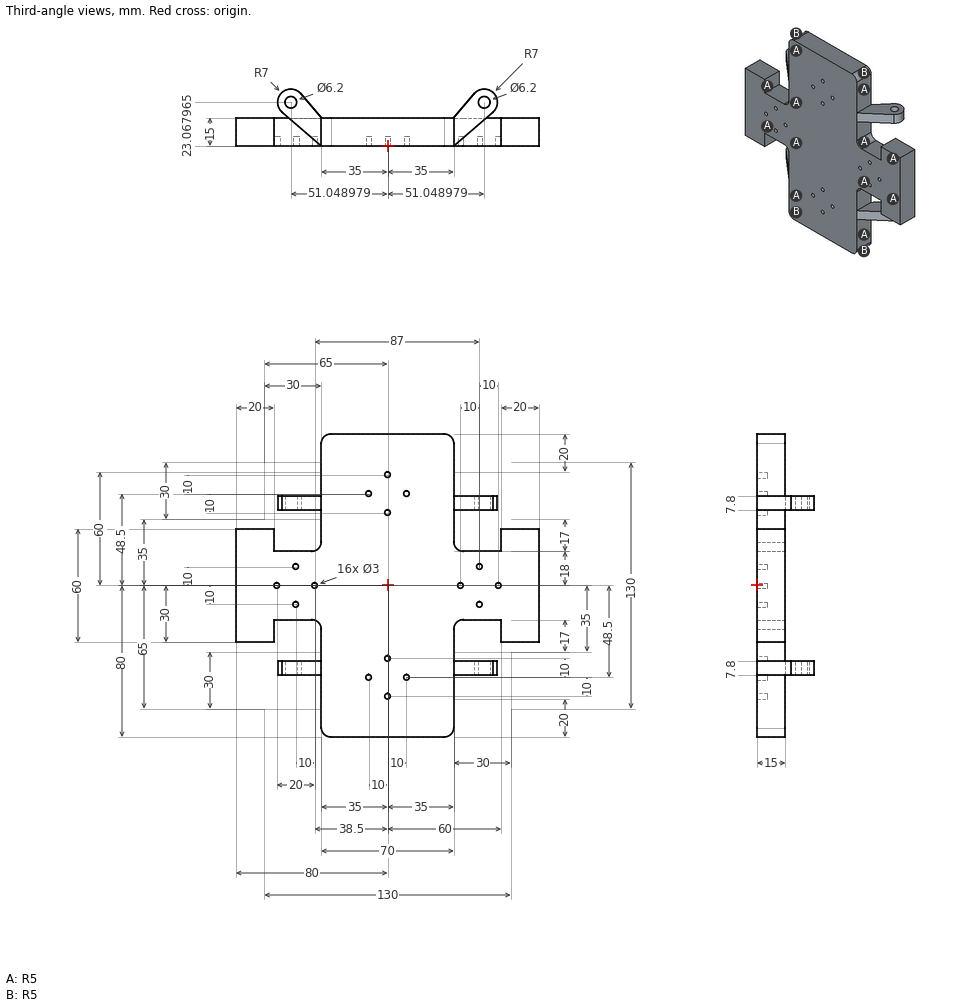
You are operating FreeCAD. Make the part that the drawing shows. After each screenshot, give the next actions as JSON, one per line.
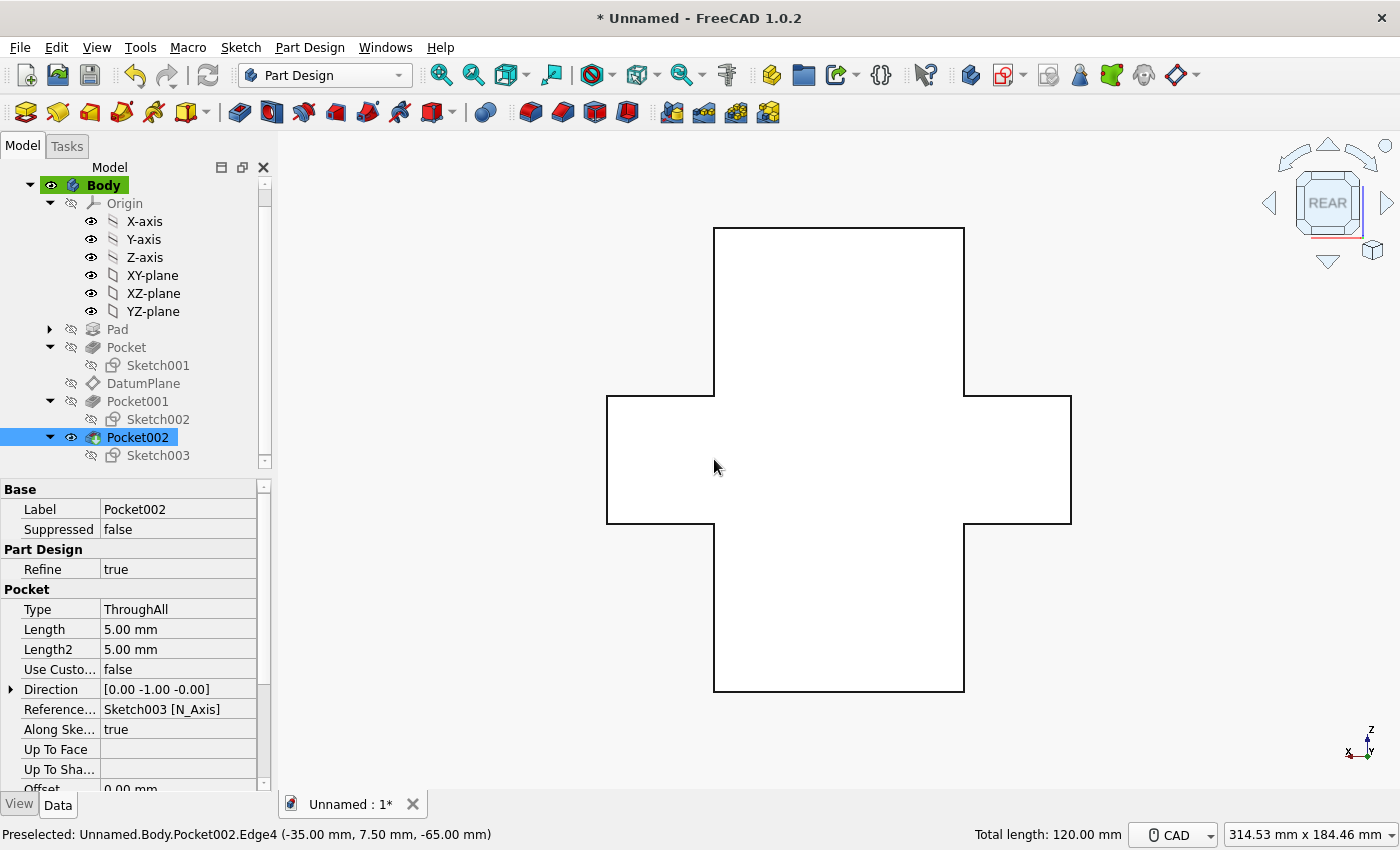
{"action": "key", "text": "6"}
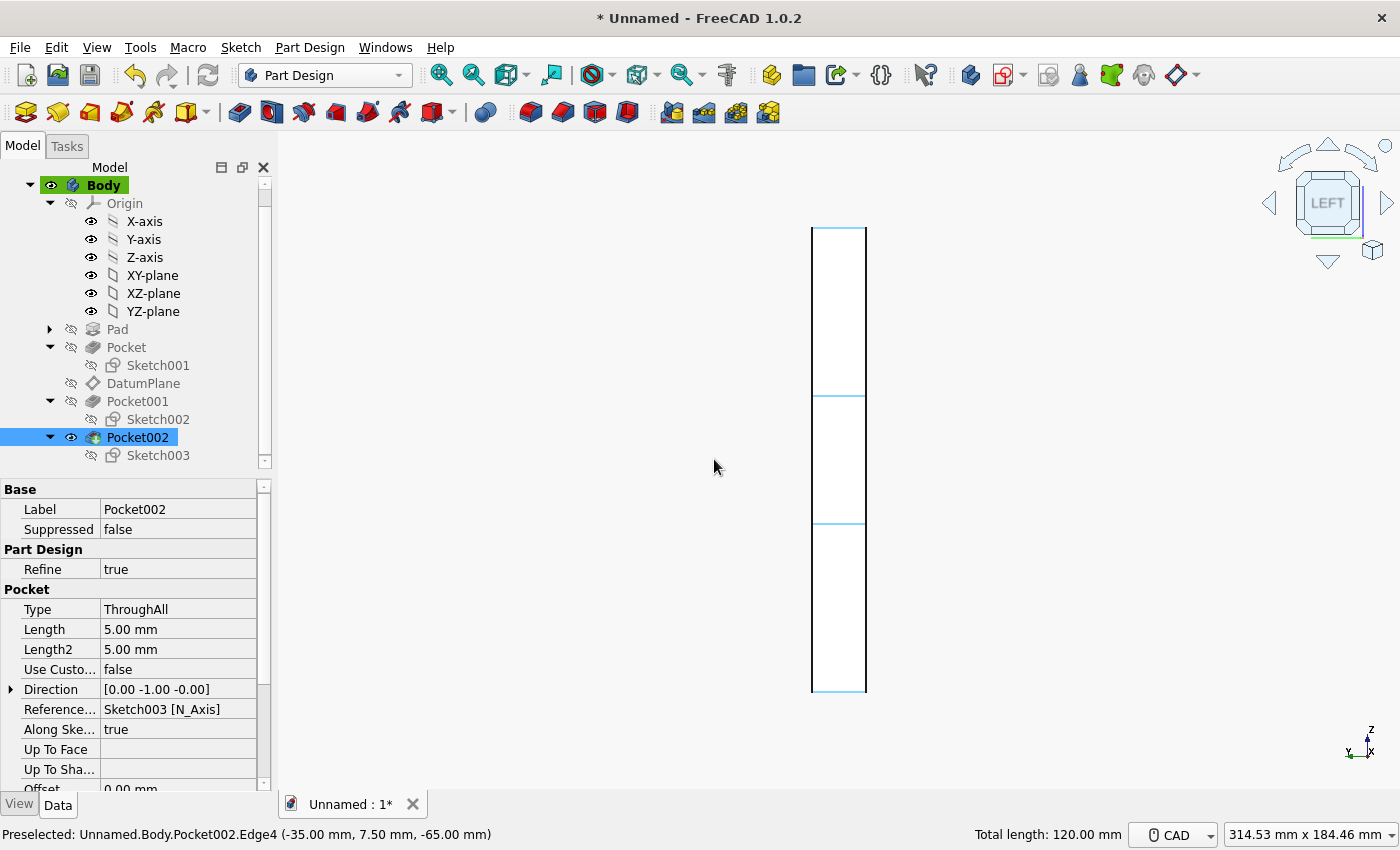
{"action": "key", "text": "v 3"}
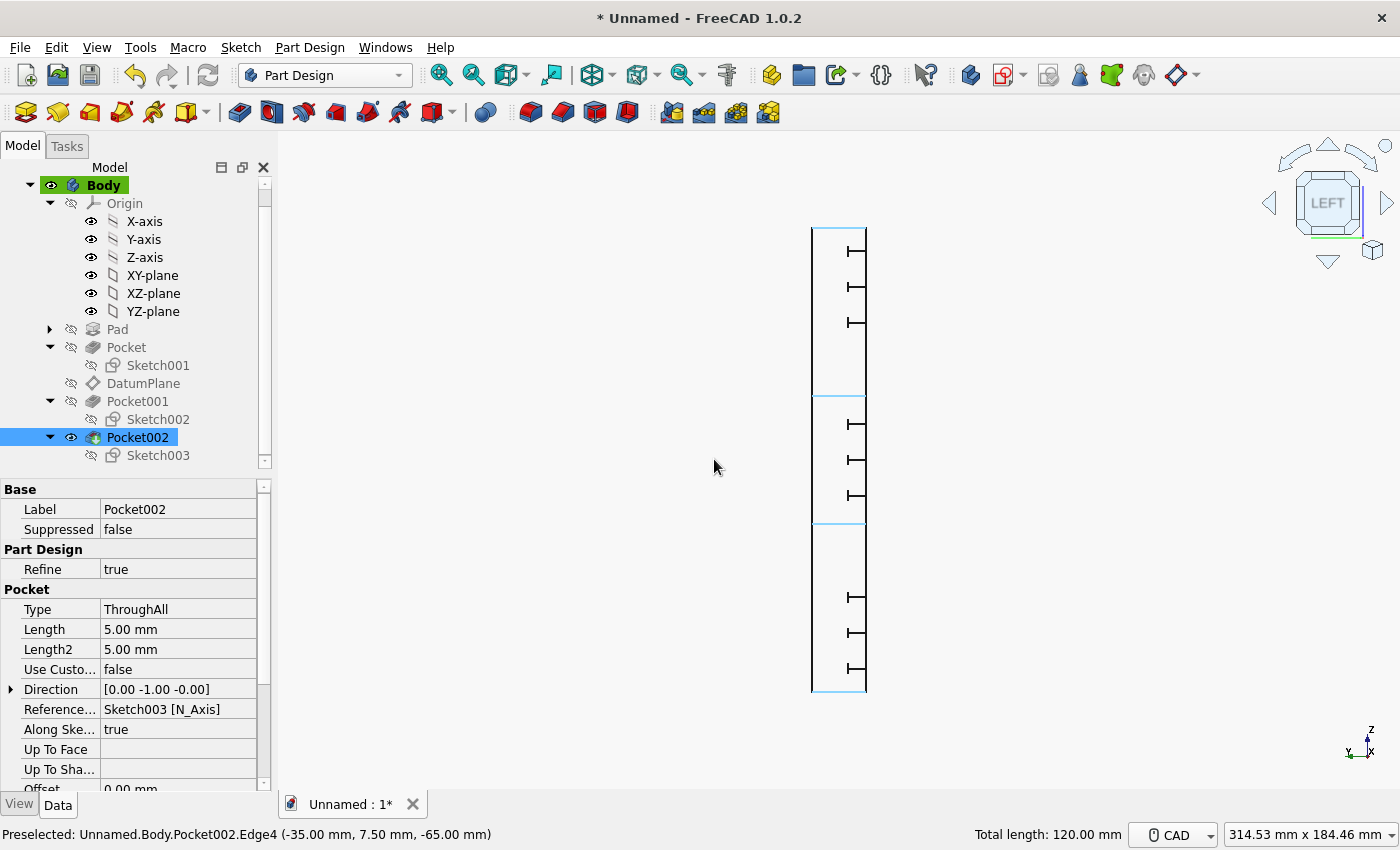
{"action": "key", "text": "0"}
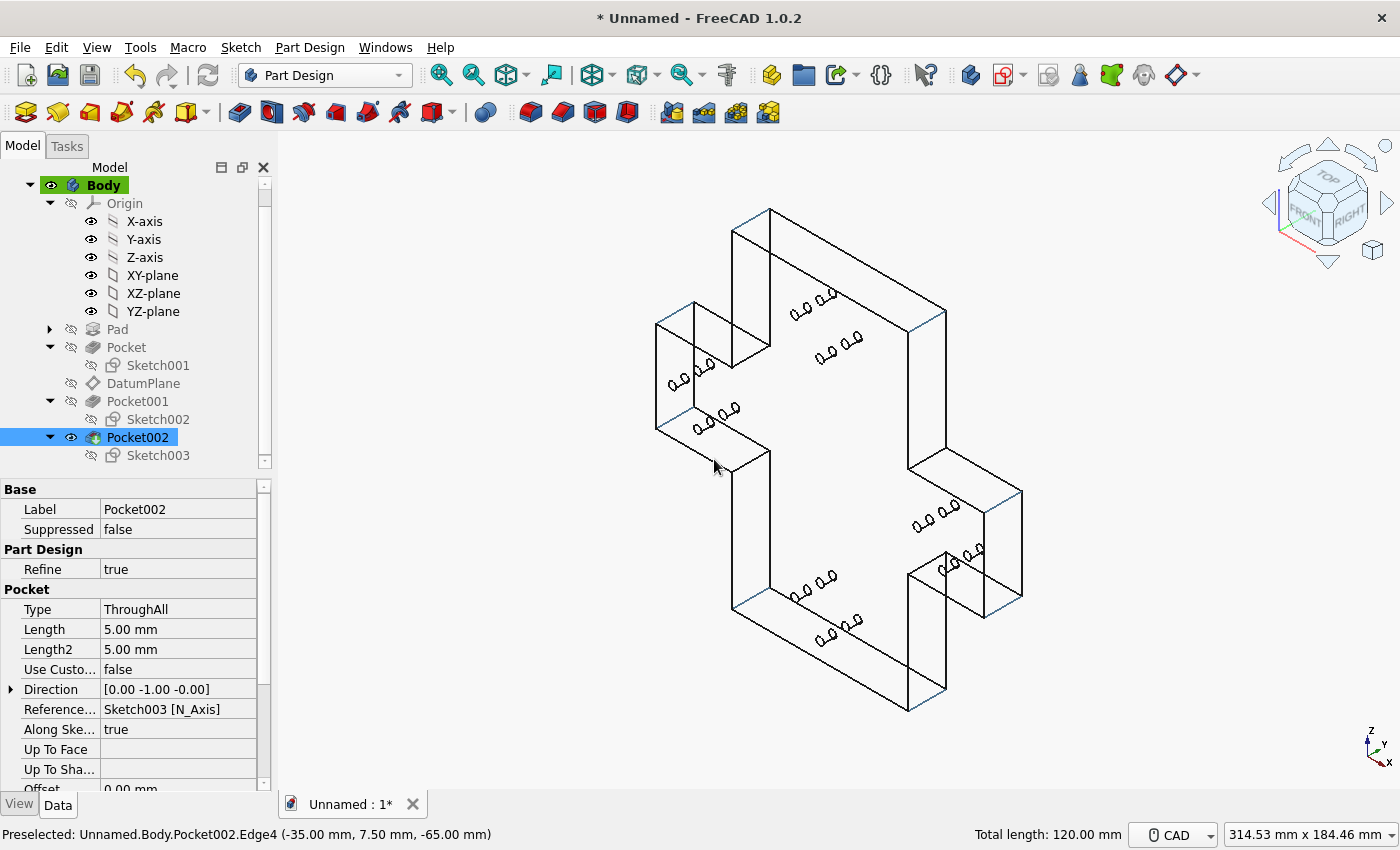
{"action": "left_click", "coordinate": [927, 458], "text": "ctrl"}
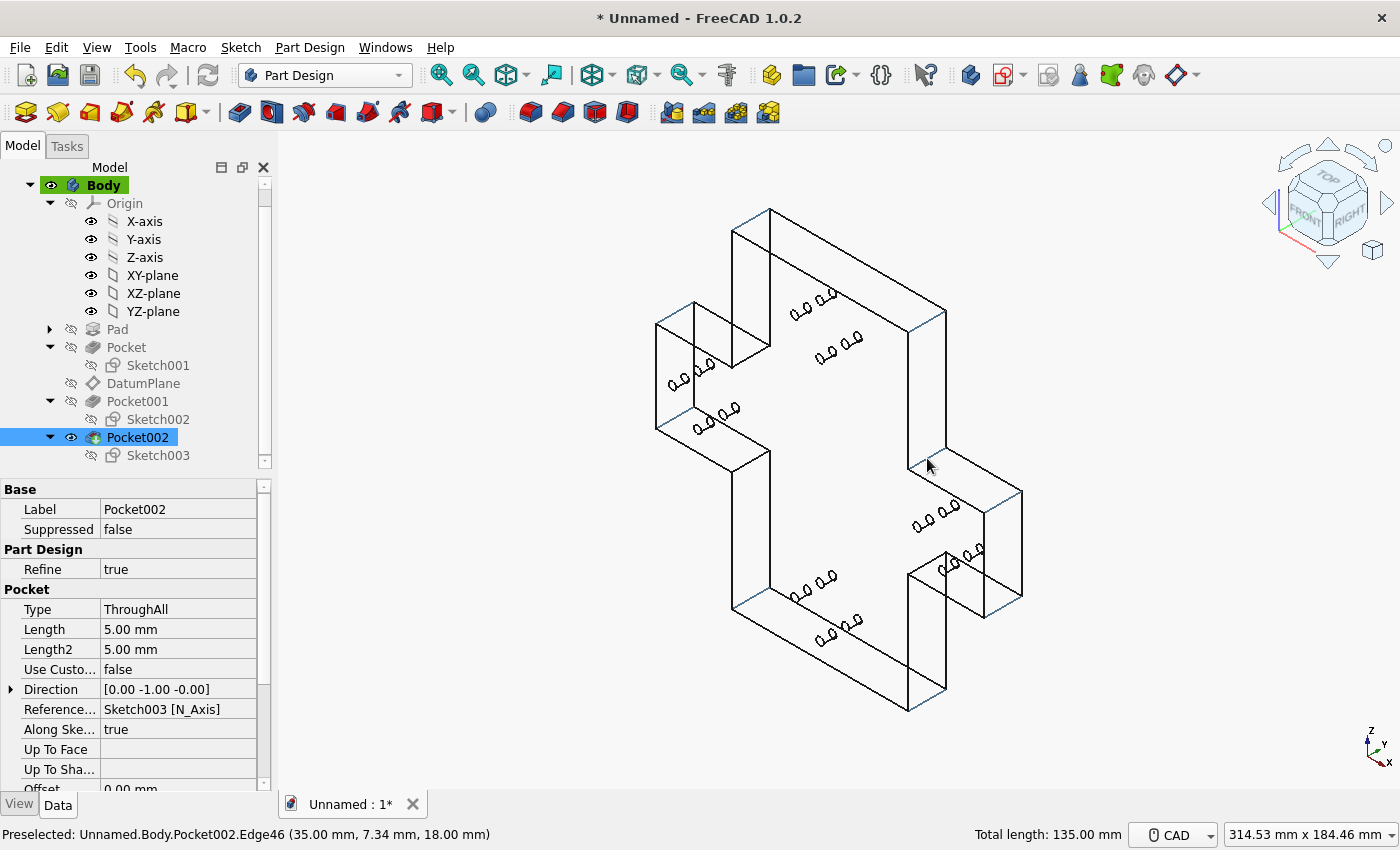
{"action": "left_click", "coordinate": [751, 460], "text": "ctrl"}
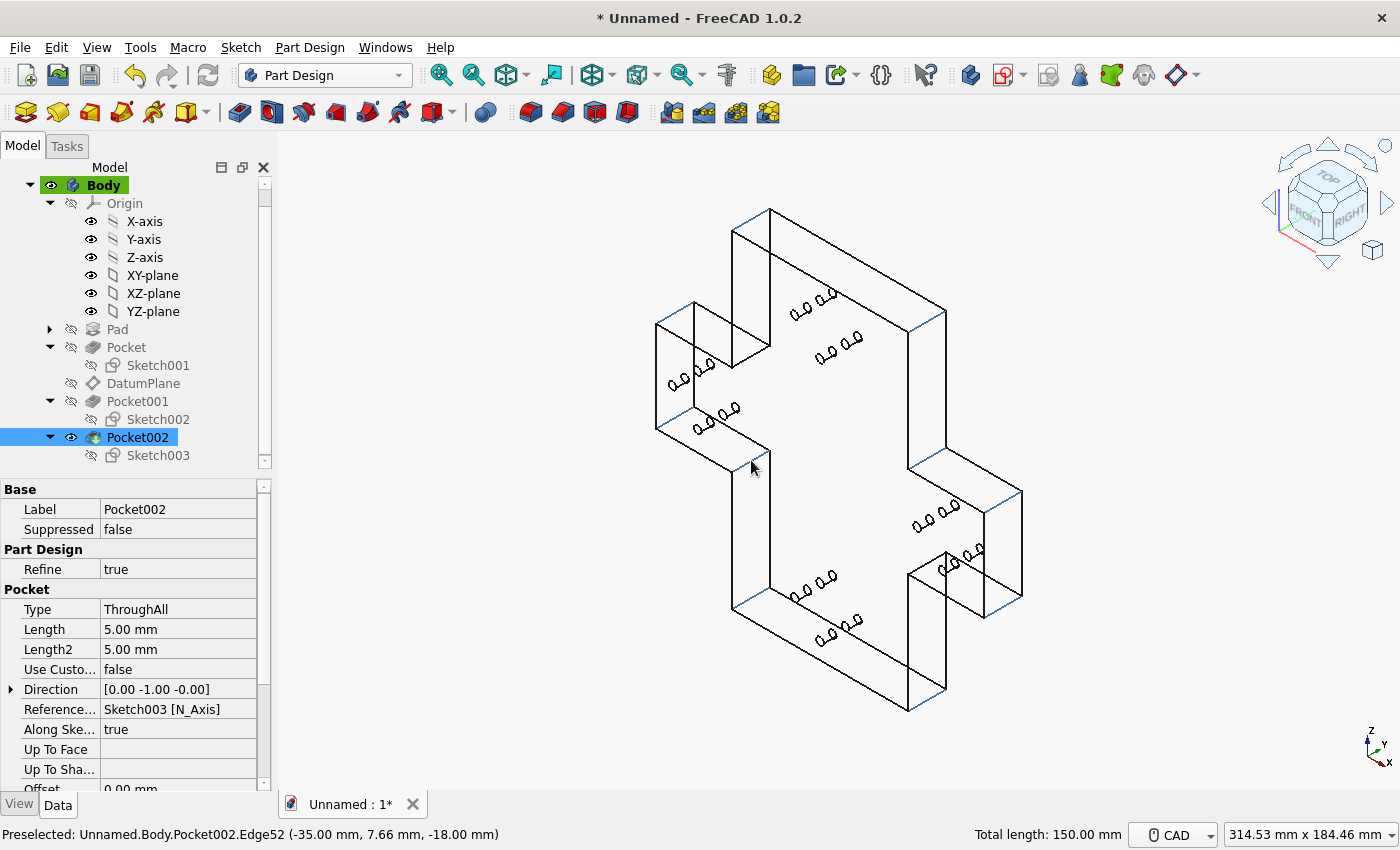
{"action": "left_click", "coordinate": [751, 356], "text": "ctrl"}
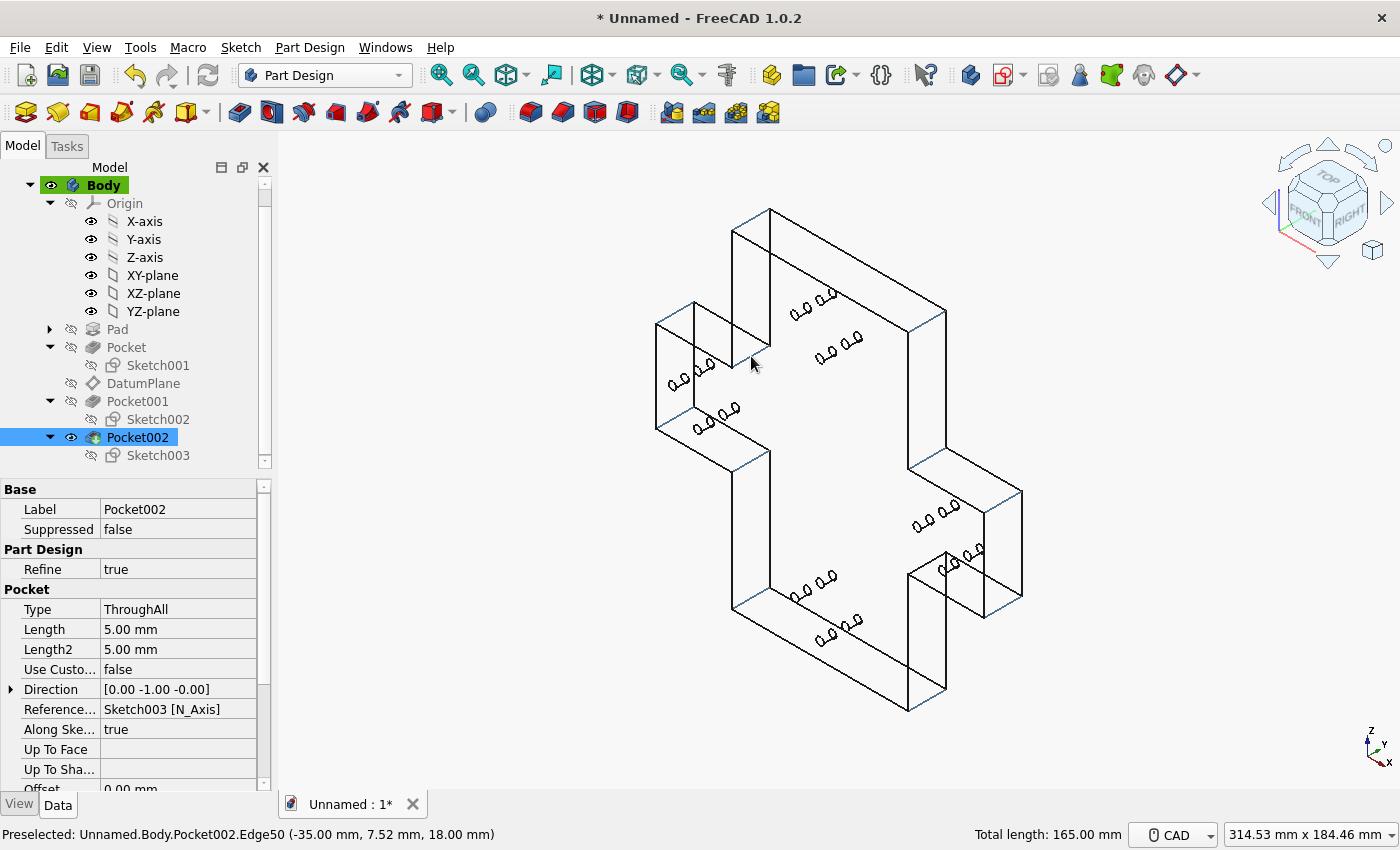
{"action": "left_click", "coordinate": [927, 562], "text": "ctrl"}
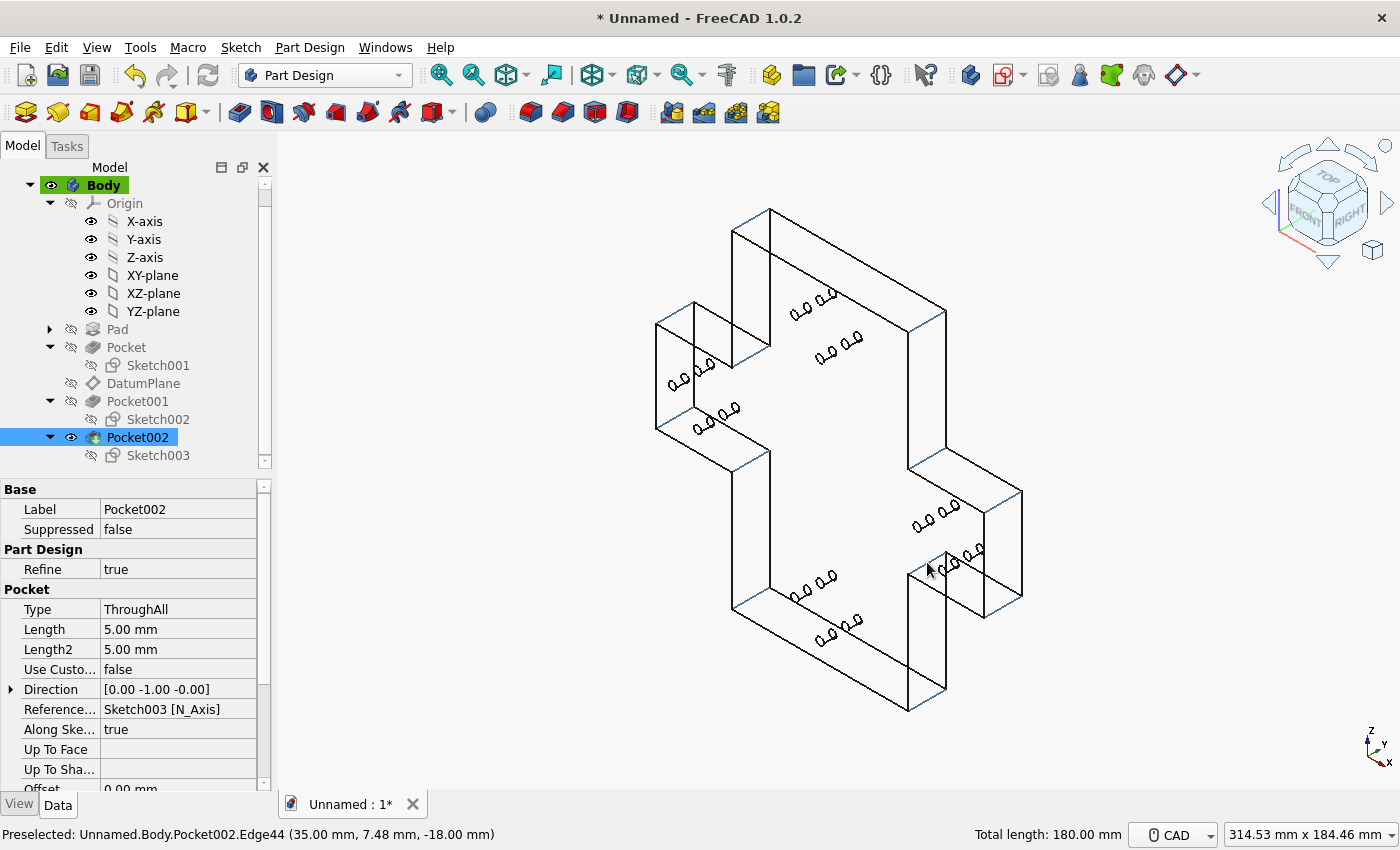
{"action": "key", "text": "v 1"}